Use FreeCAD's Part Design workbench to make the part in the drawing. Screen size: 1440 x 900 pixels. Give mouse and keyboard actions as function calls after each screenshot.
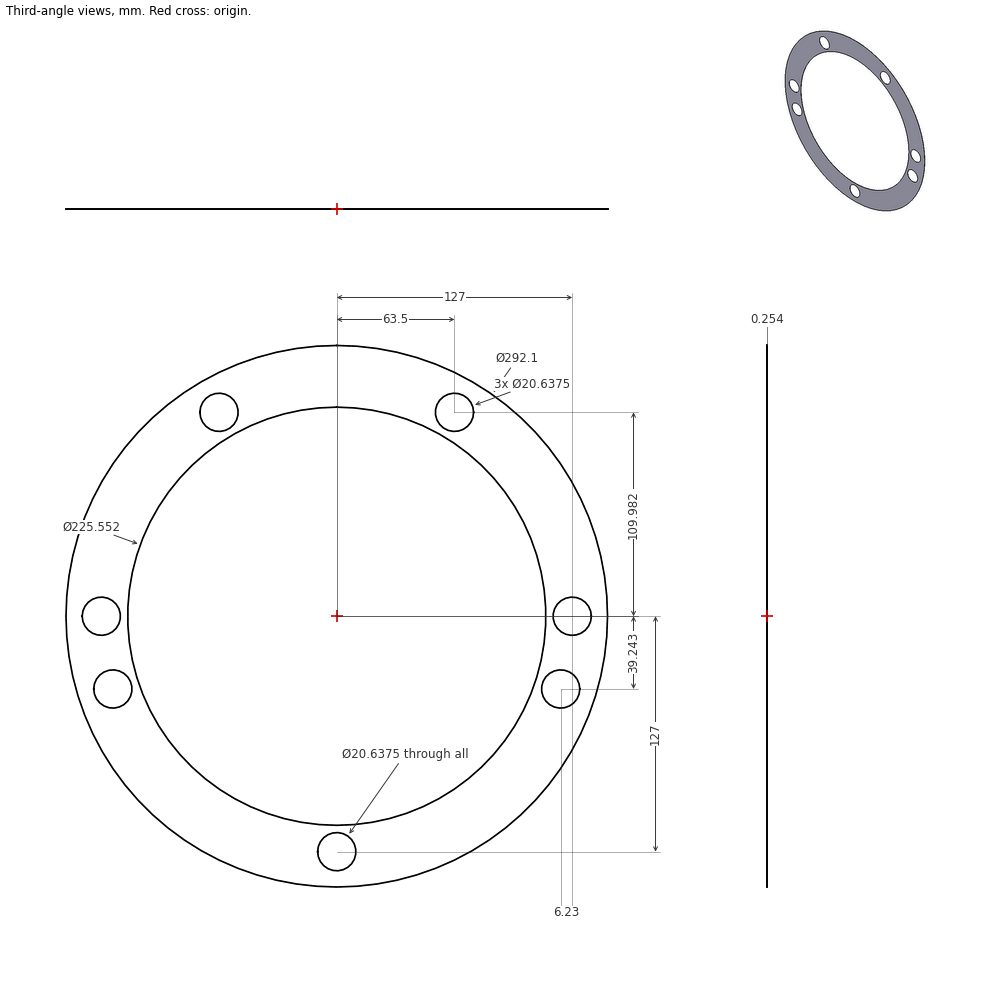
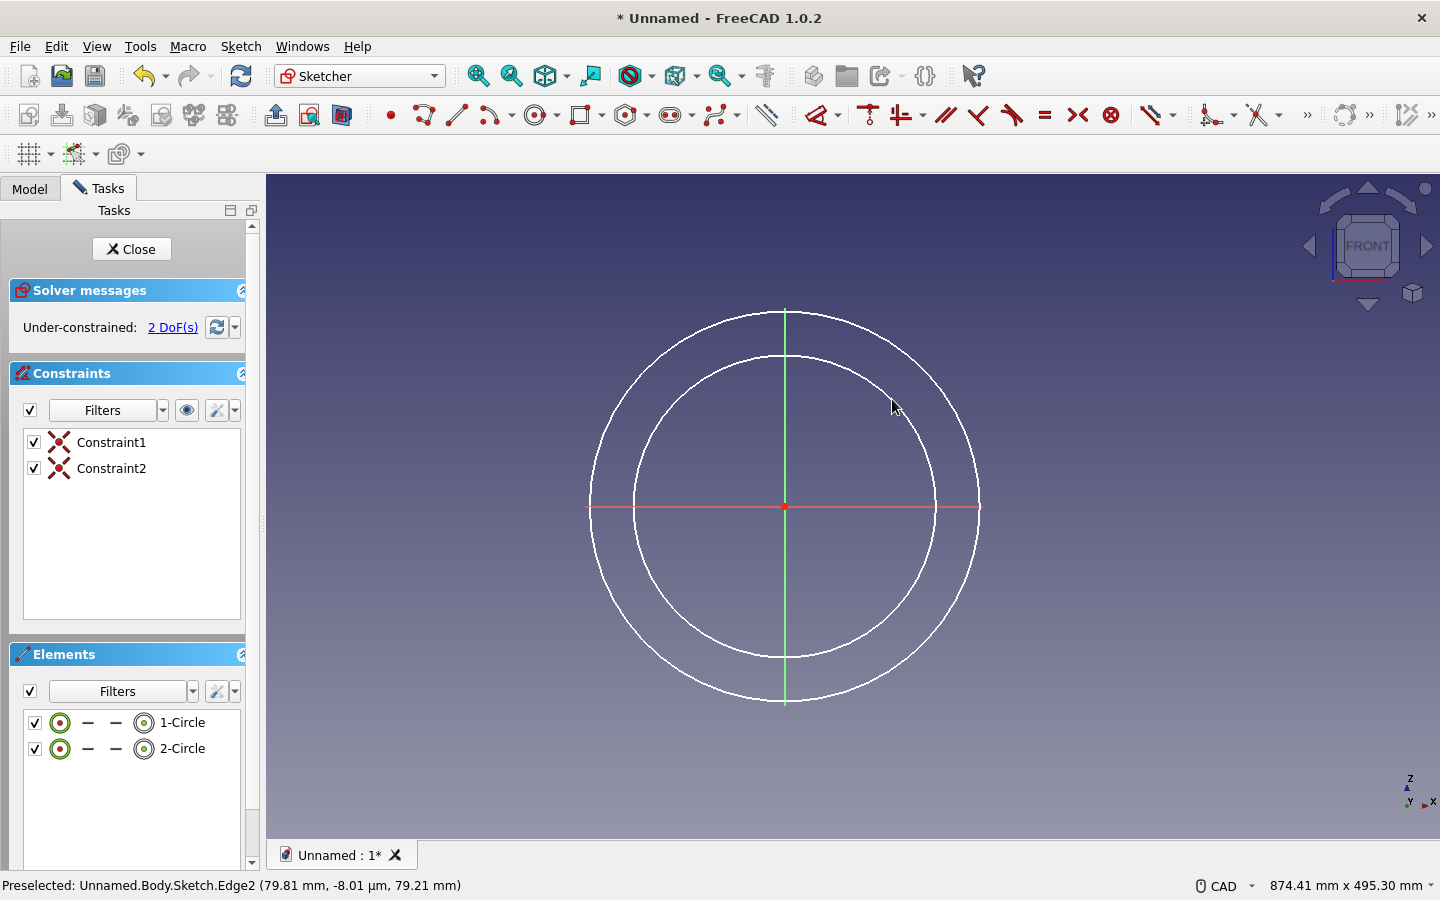
click(922, 368)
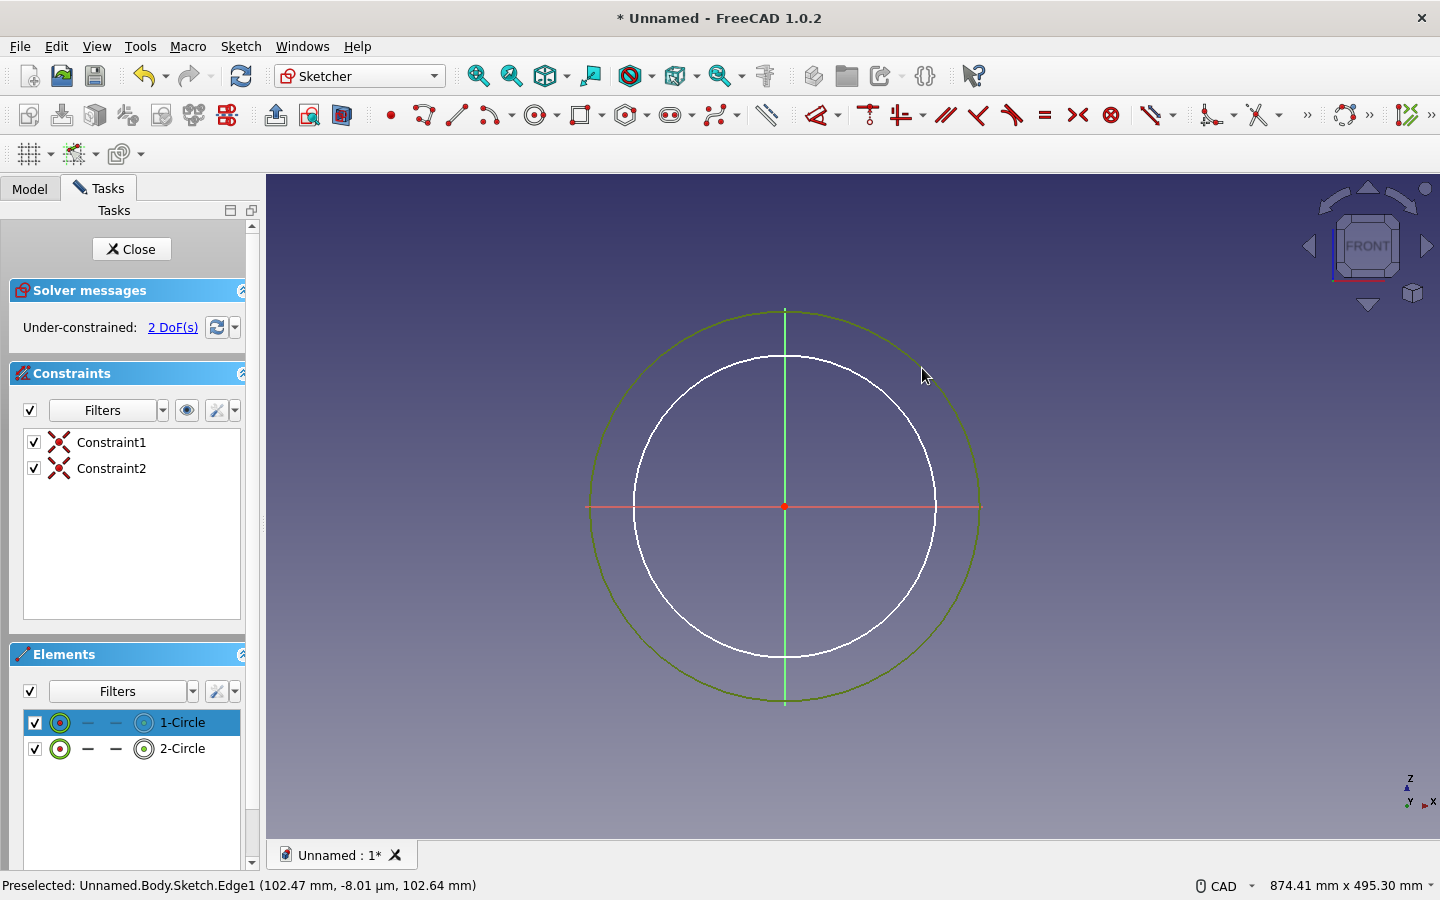
key(k)
key(o)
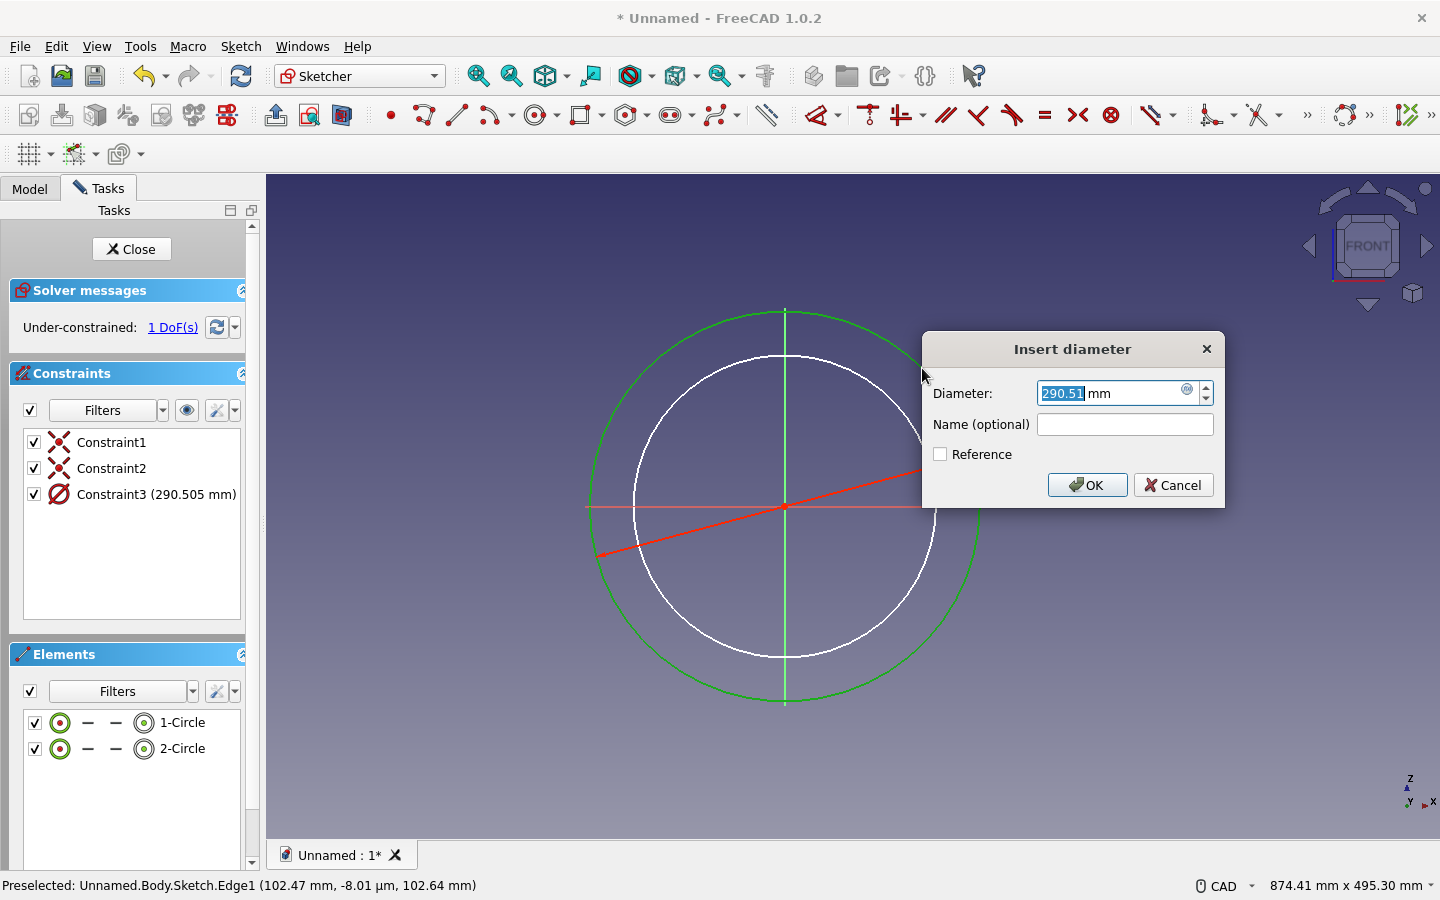
text(292.1)
key(Return)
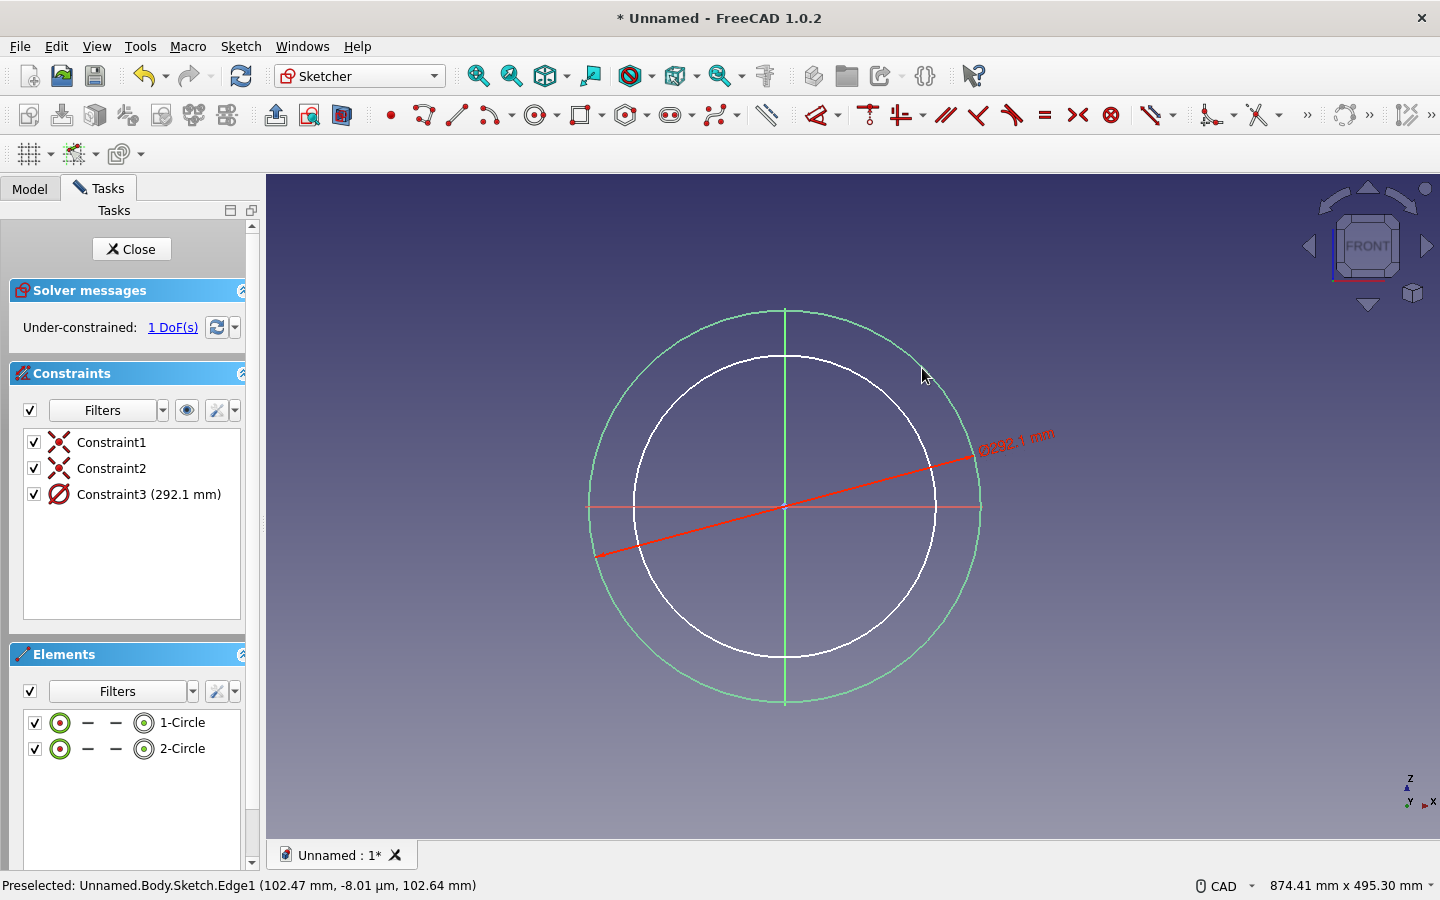
click(891, 399)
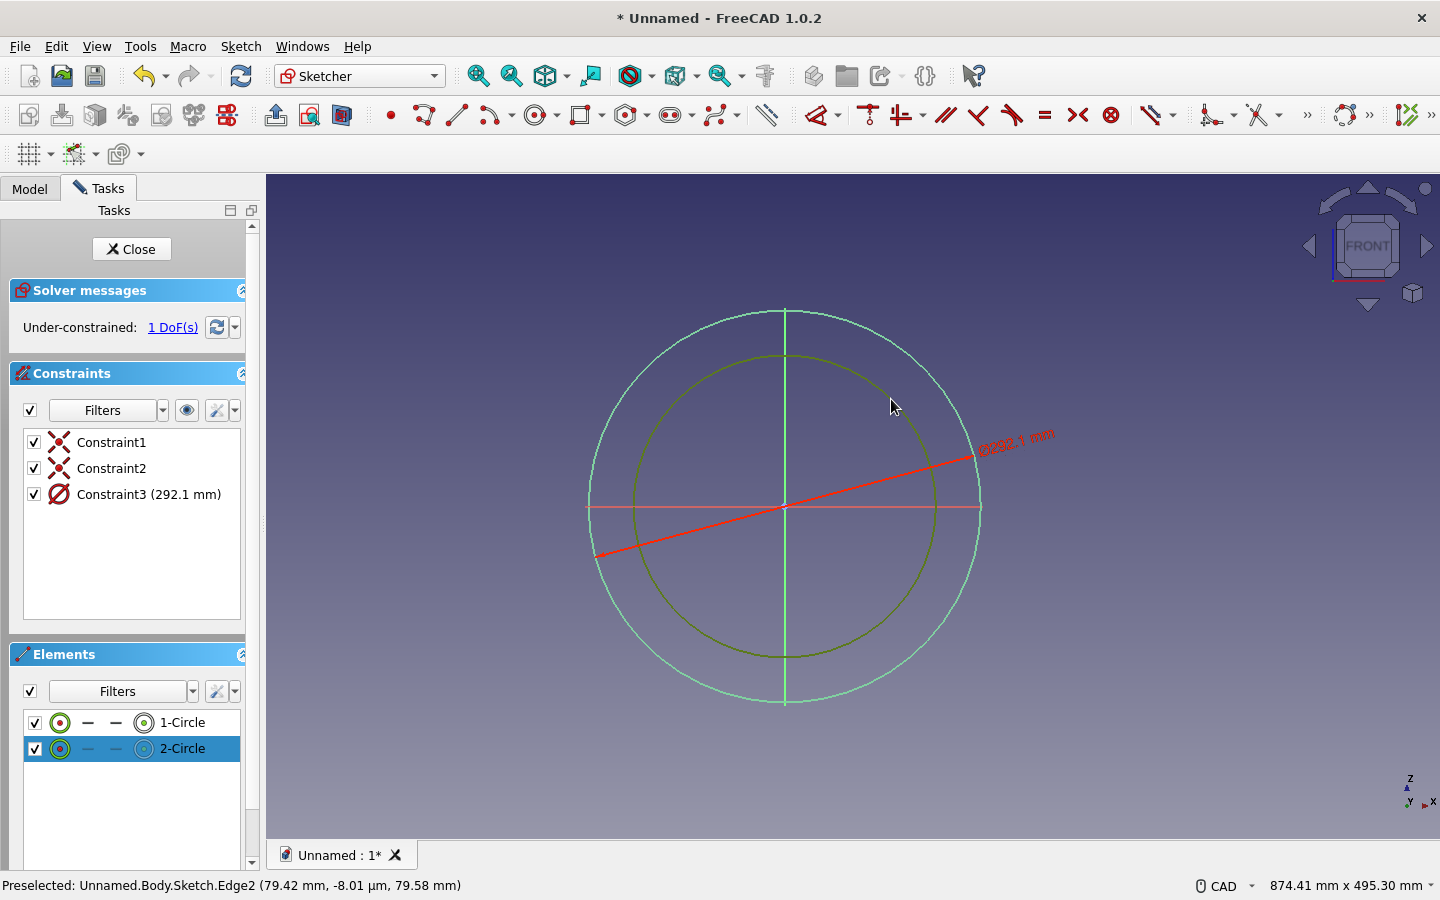
click(838, 116)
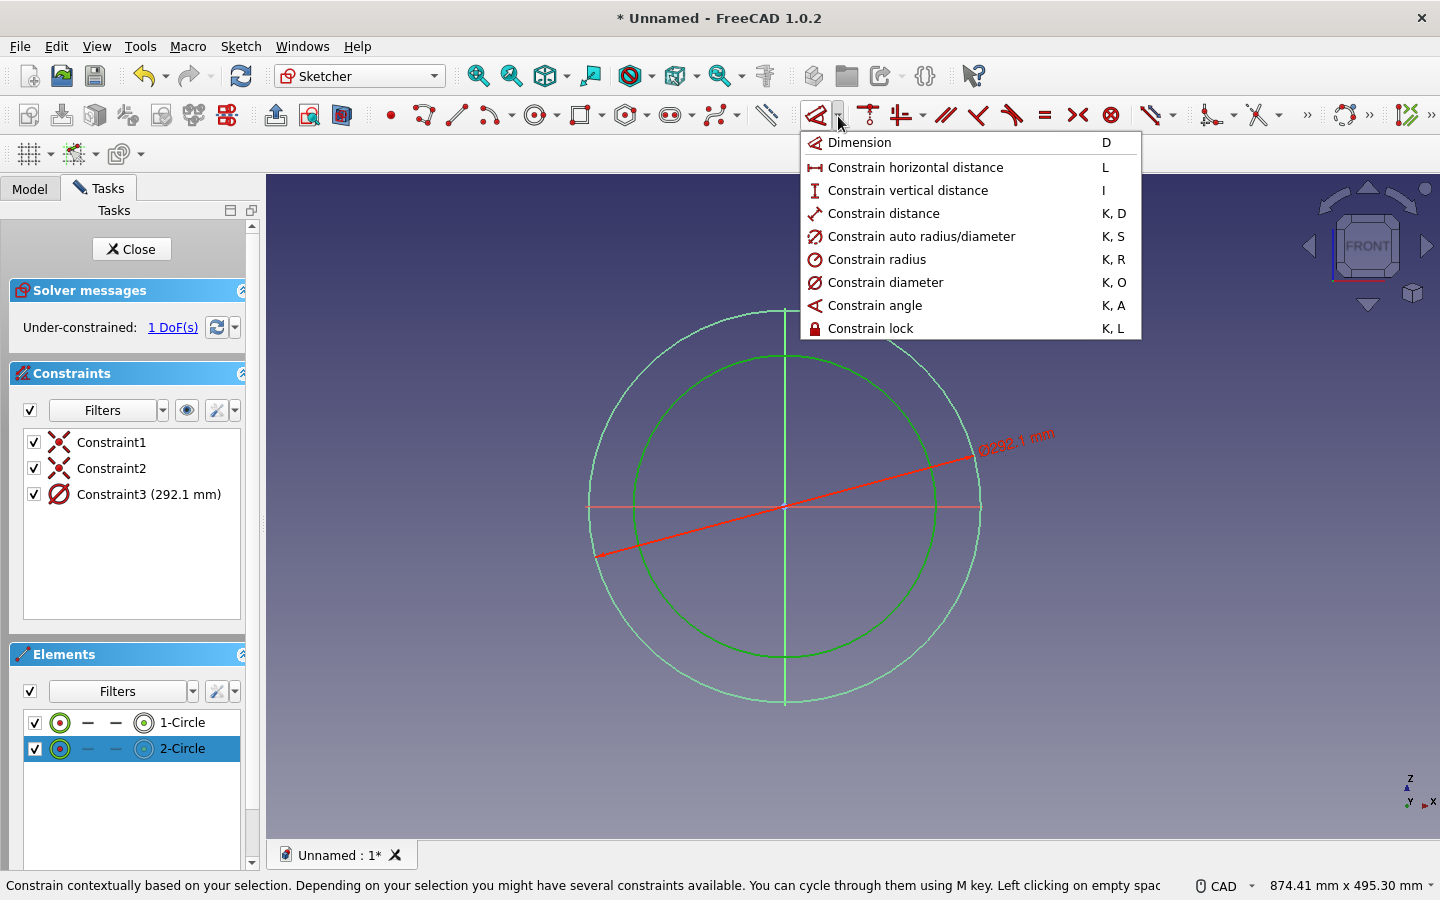
click(971, 282)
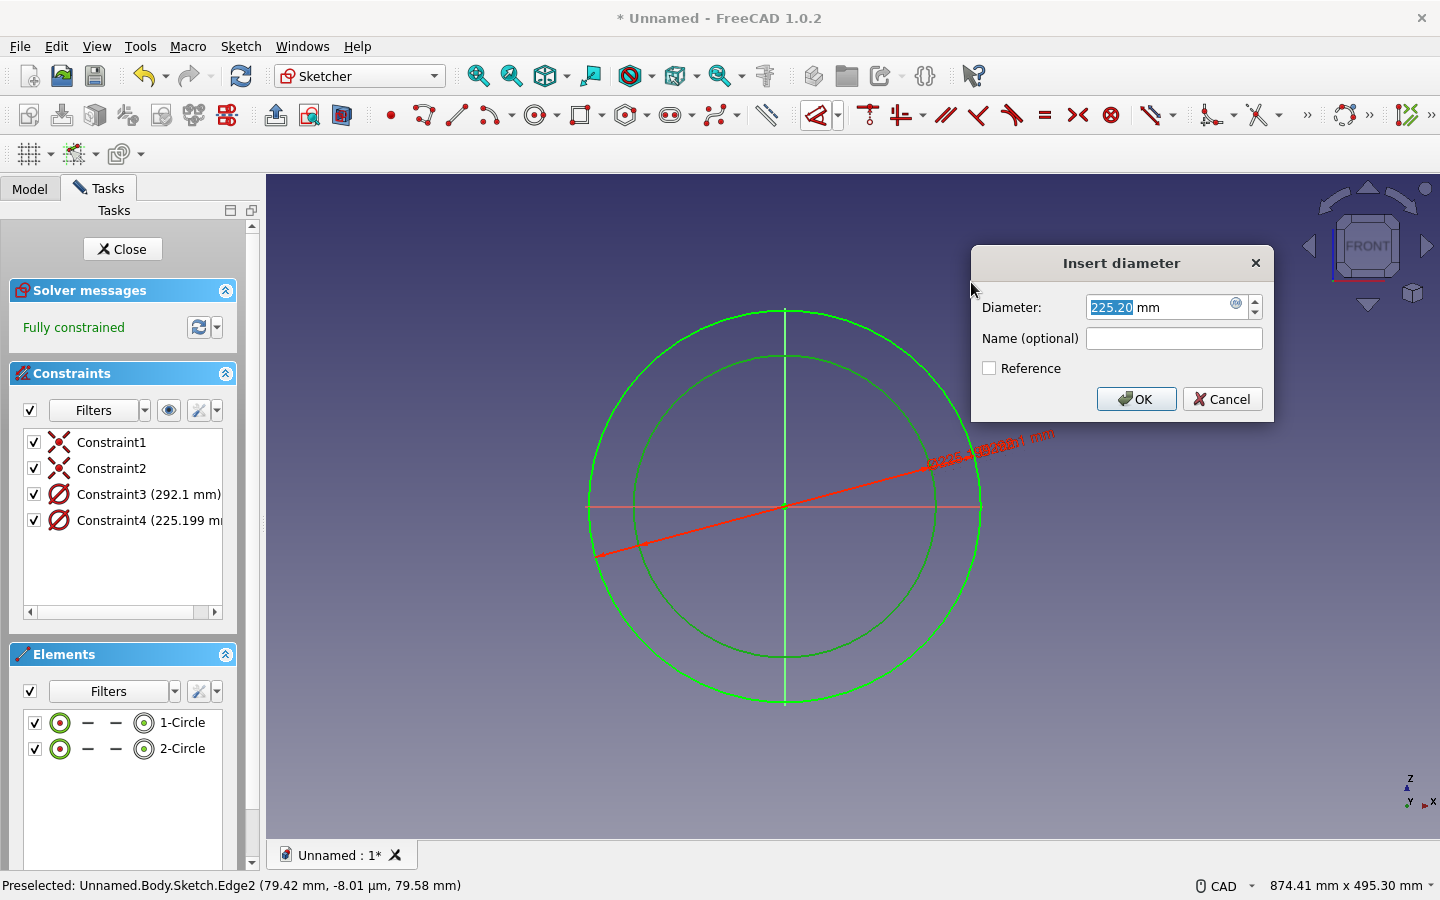
text(225.552)
key(Return)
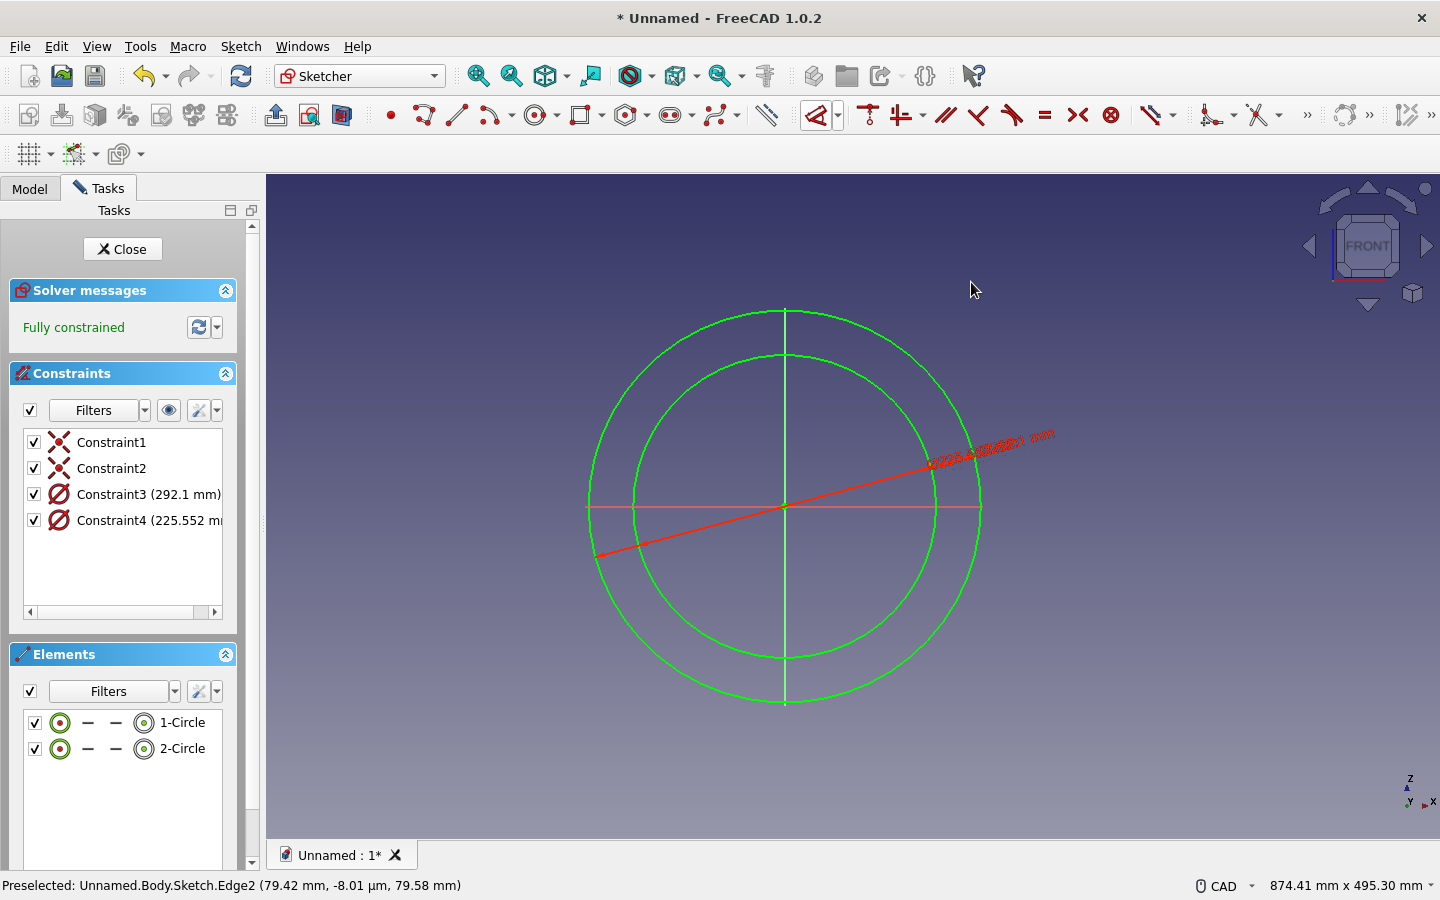
click(123, 249)